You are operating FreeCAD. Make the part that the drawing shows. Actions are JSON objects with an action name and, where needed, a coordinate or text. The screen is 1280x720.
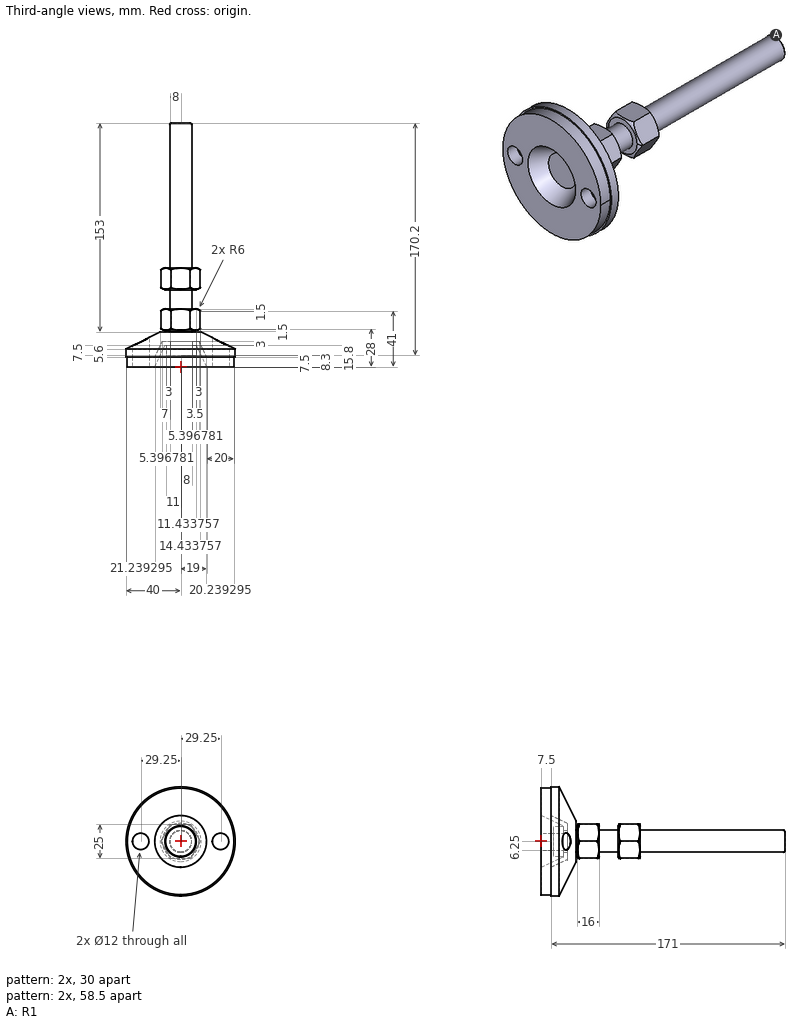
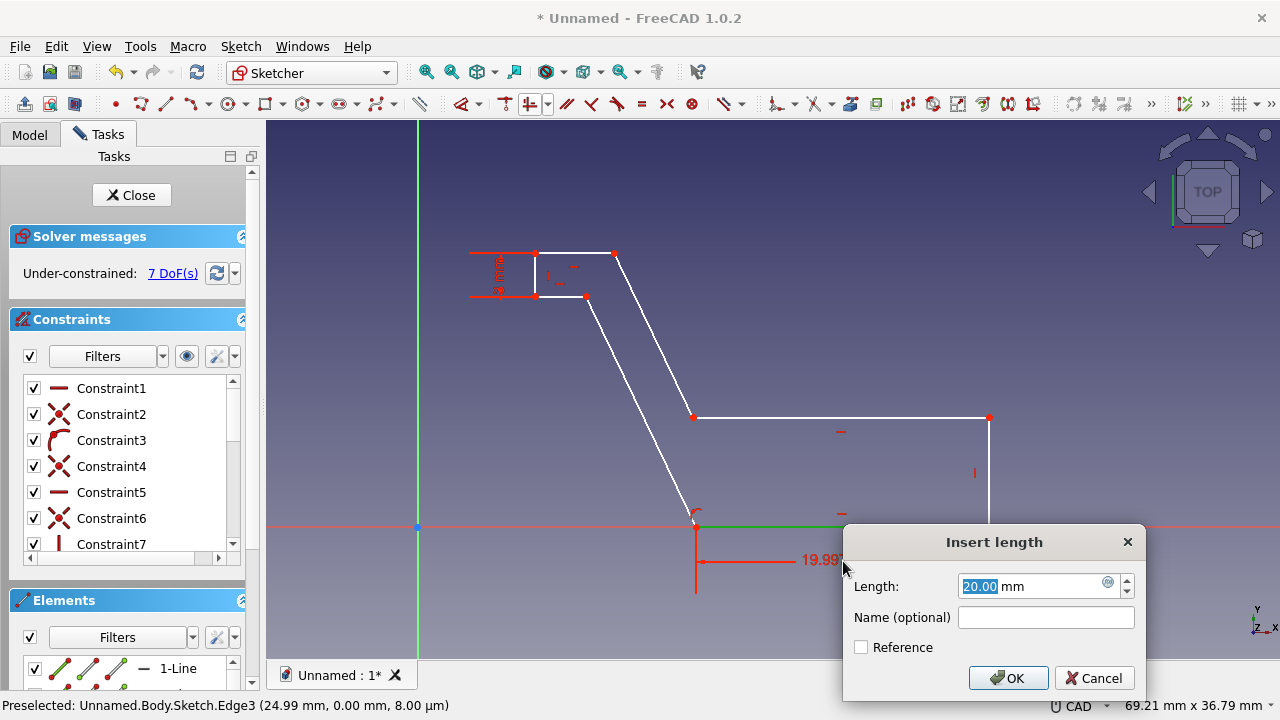
{"action": "type", "text": "20"}
{"action": "key", "text": "Return"}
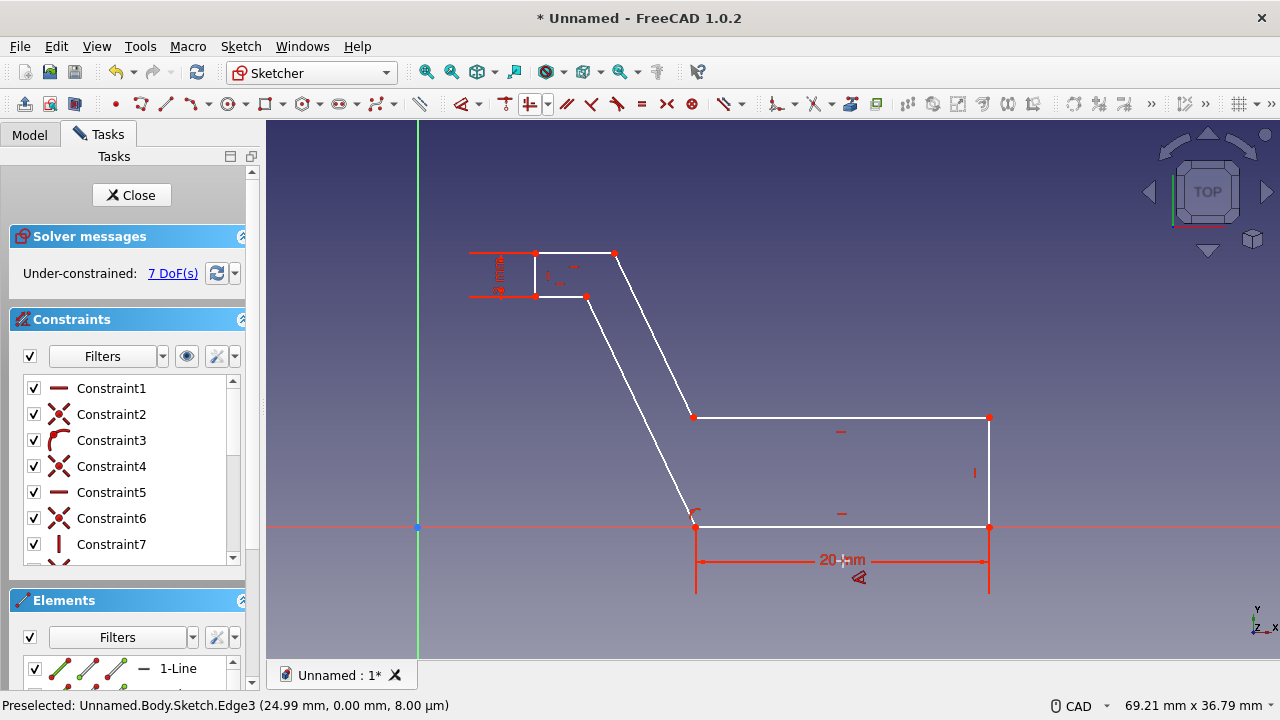
{"action": "left_click", "coordinate": [535, 297]}
{"action": "left_click", "coordinate": [476, 561]}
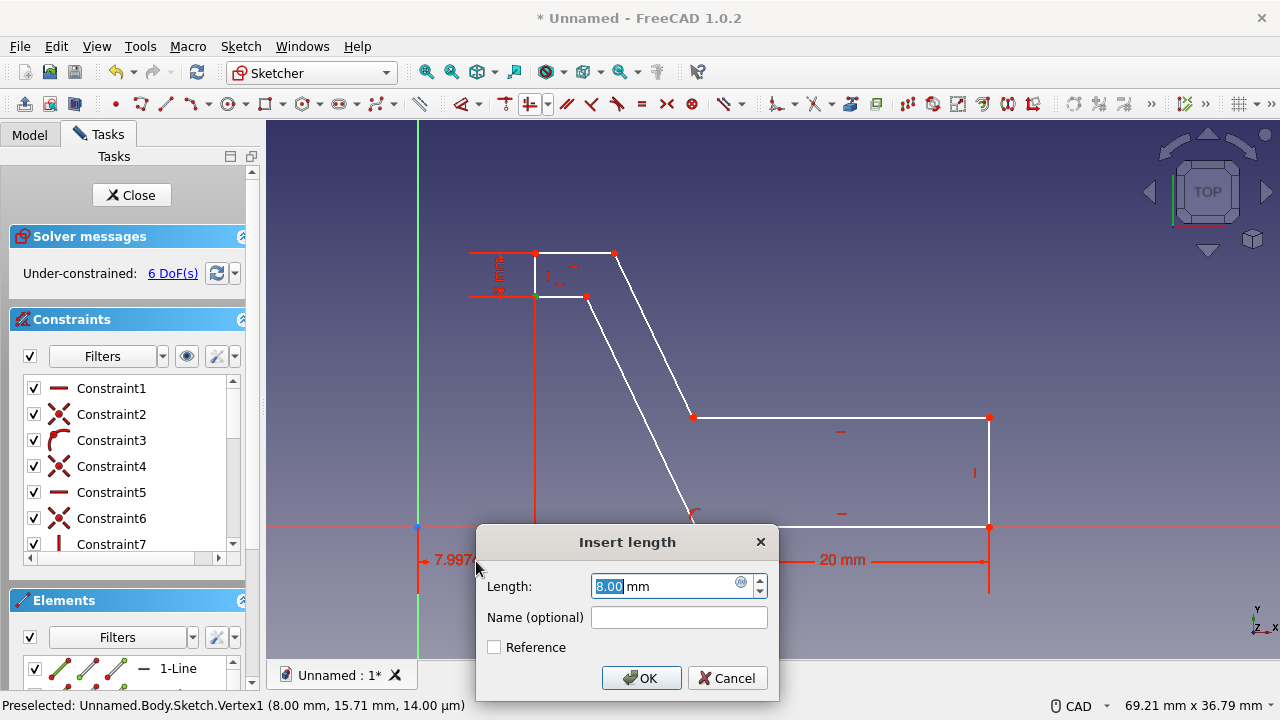
{"action": "type", "text": "8"}
{"action": "key", "text": "Return"}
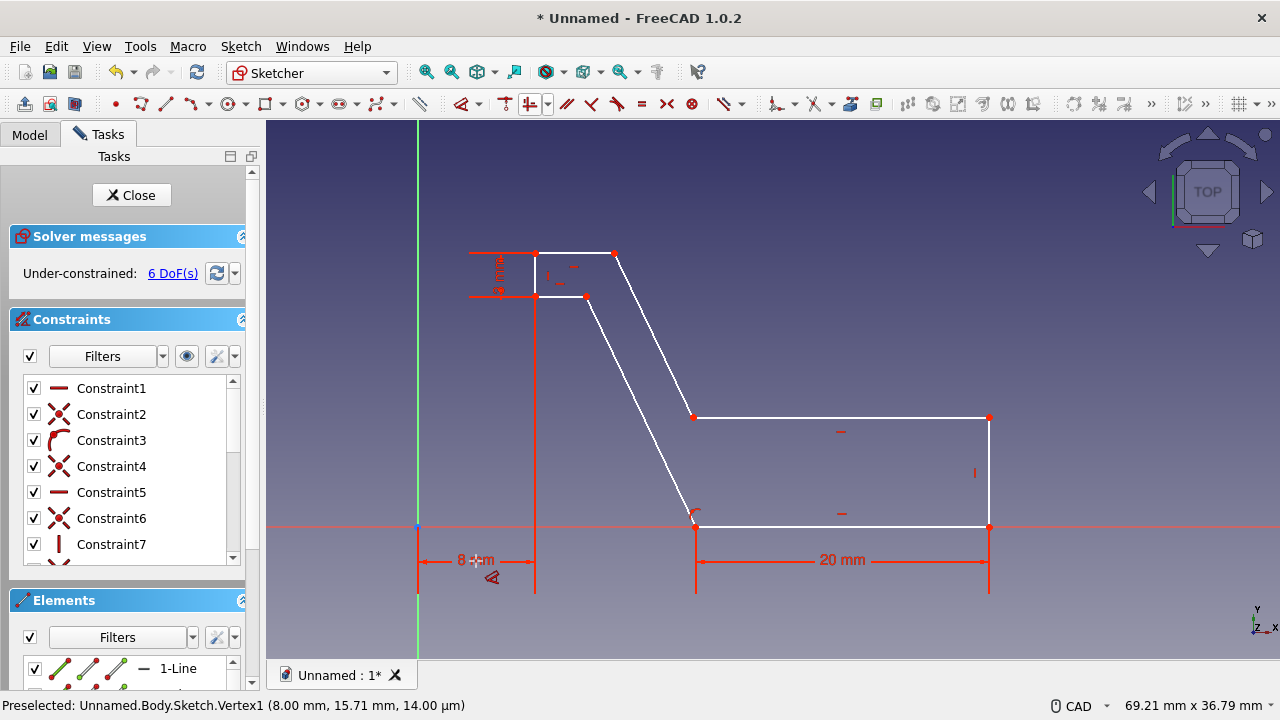
{"action": "left_click", "coordinate": [550, 297]}
{"action": "left_click", "coordinate": [561, 331]}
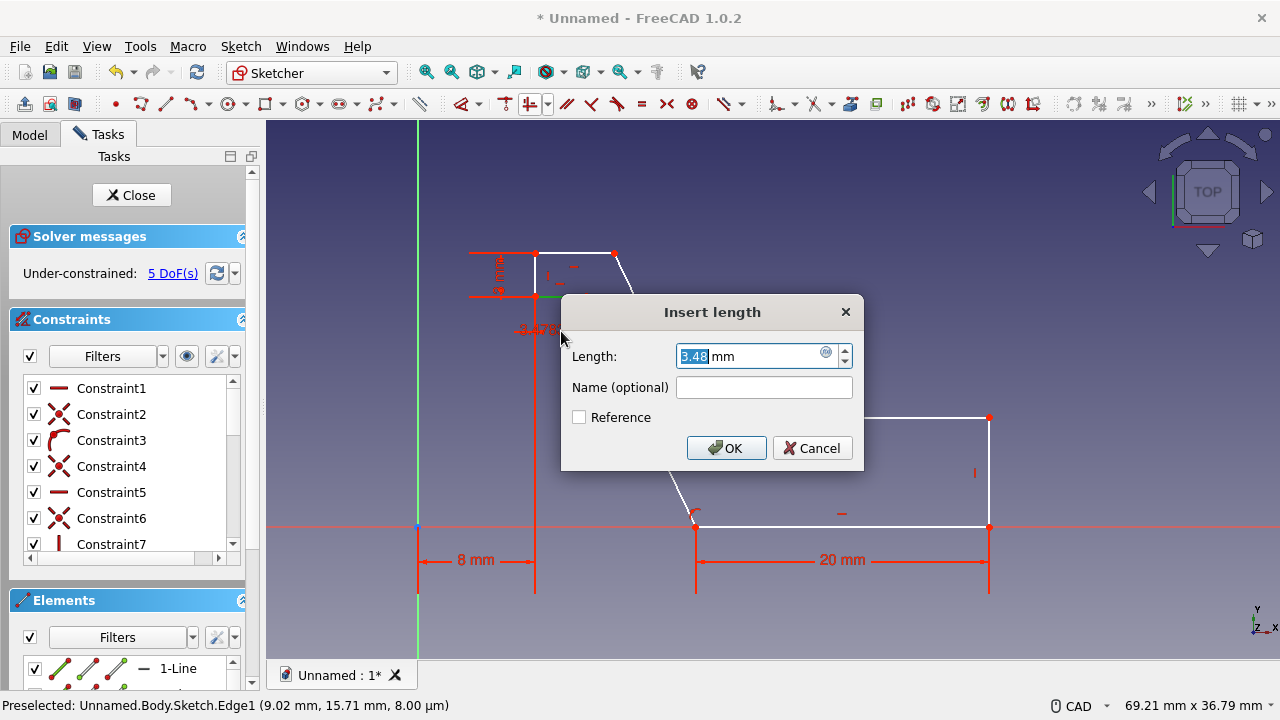
{"action": "type", "text": "3.5"}
{"action": "key", "text": "Return"}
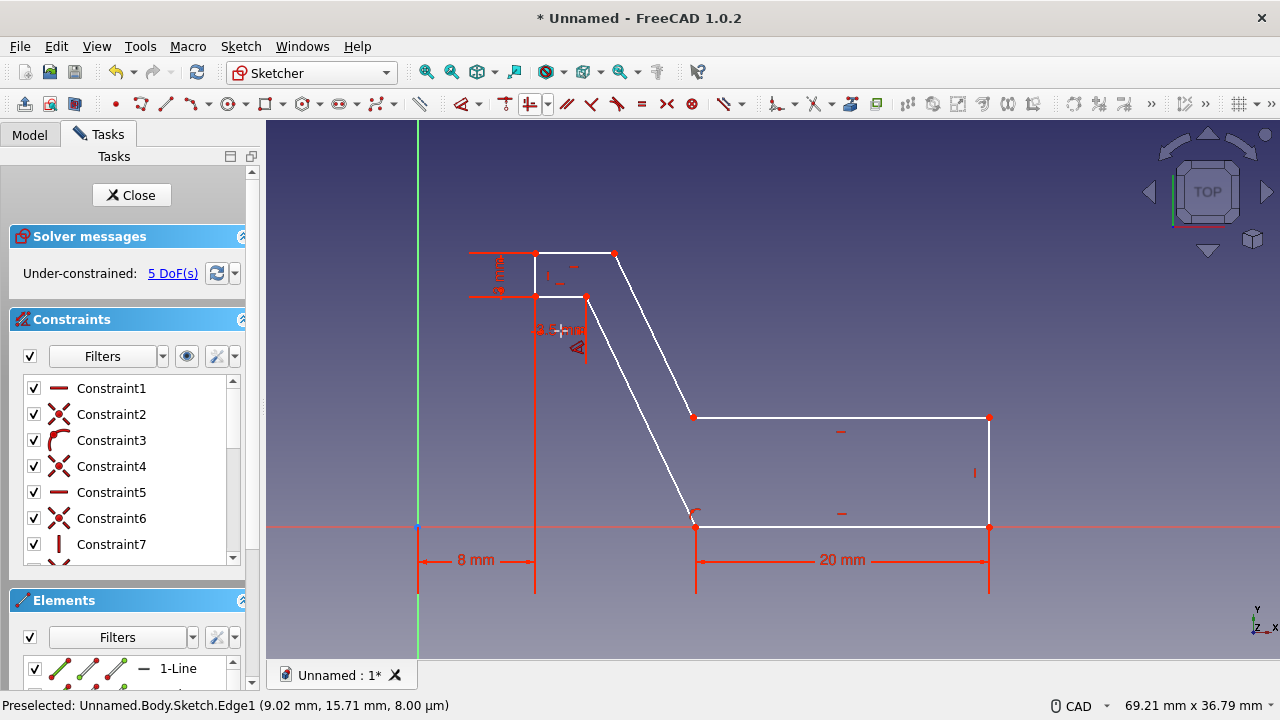
{"action": "left_click", "coordinate": [989, 494]}
{"action": "left_click", "coordinate": [1023, 473]}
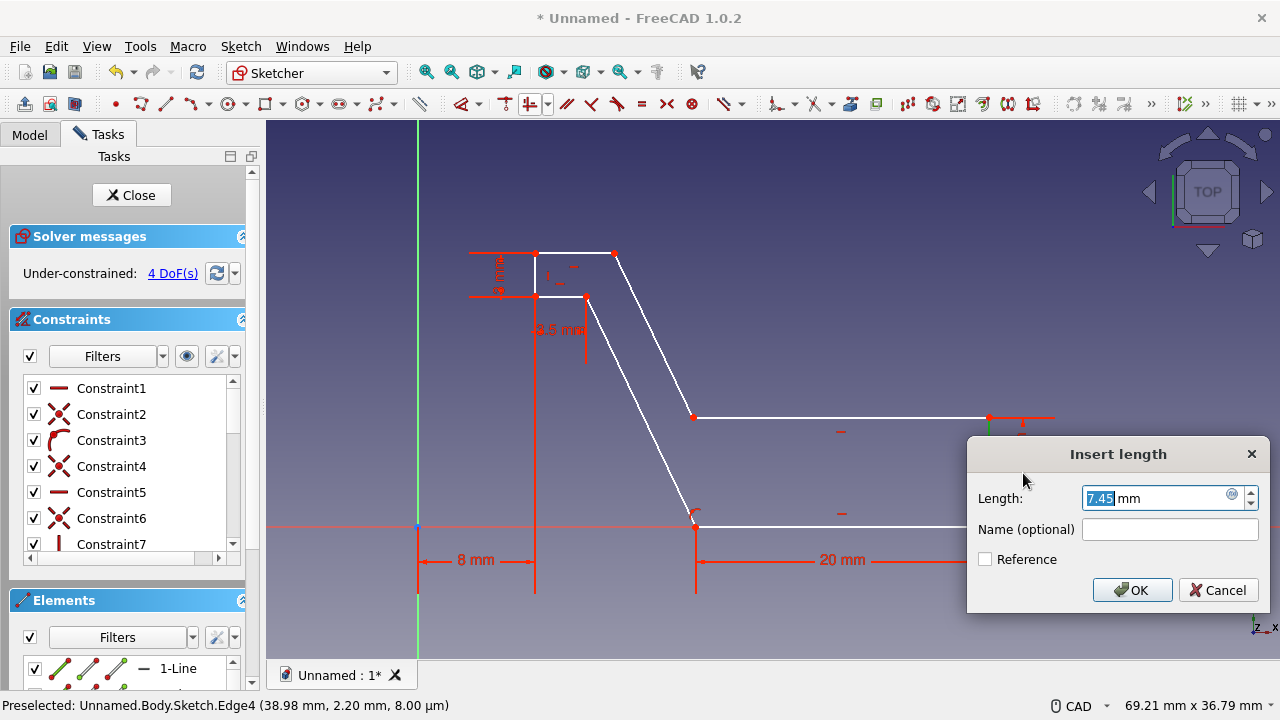
{"action": "type", "text": "7.5"}
{"action": "key", "text": "Return"}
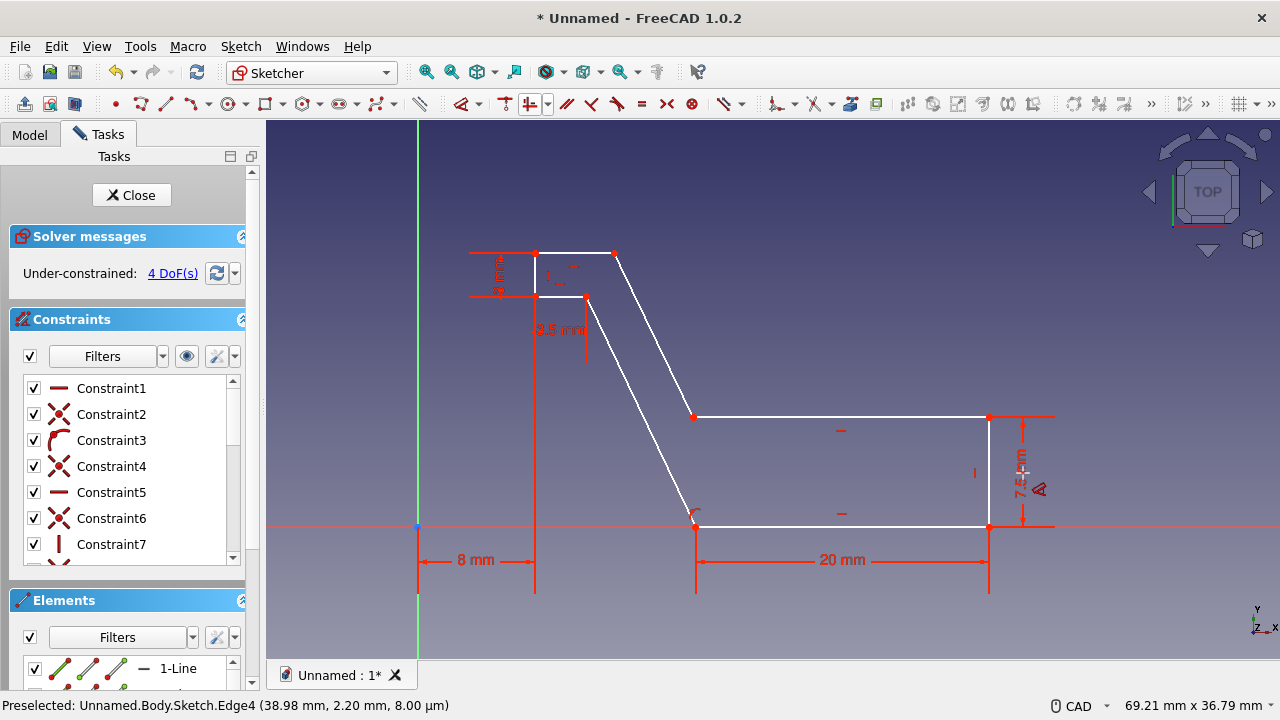
{"action": "left_click", "coordinate": [696, 527]}
{"action": "left_click", "coordinate": [557, 561]}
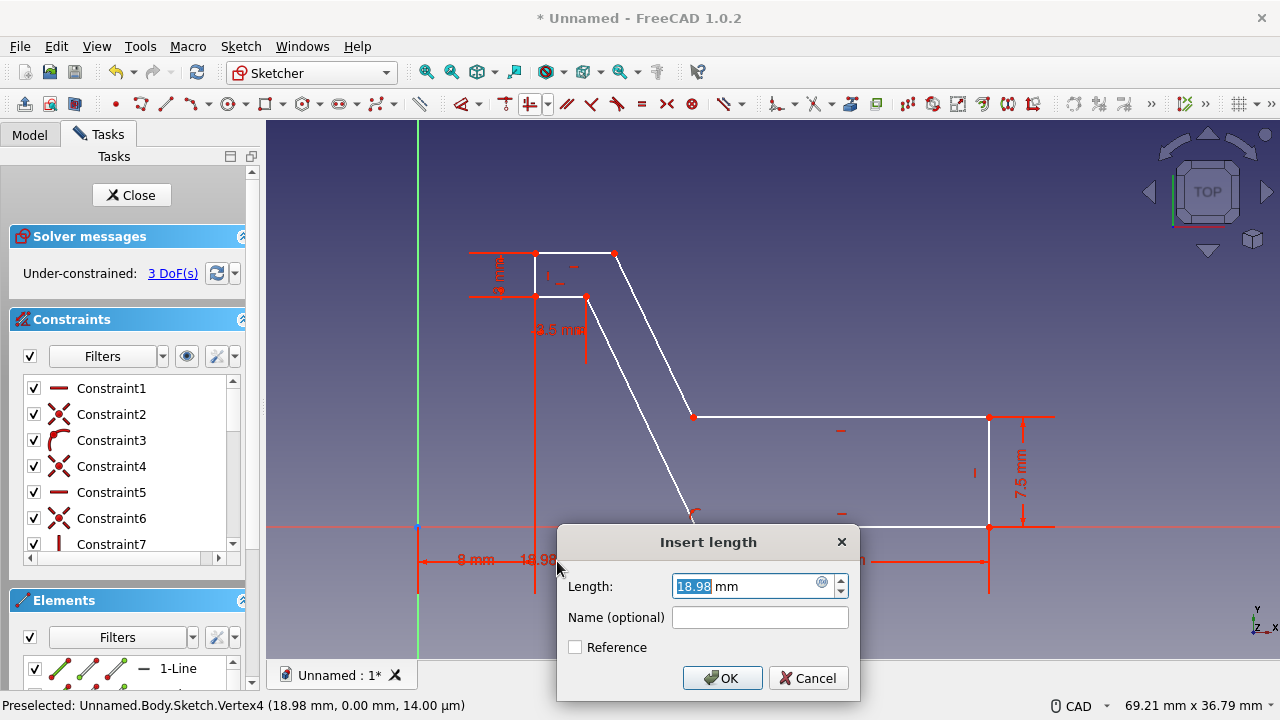
{"action": "type", "text": "19"}
{"action": "key", "text": "Return"}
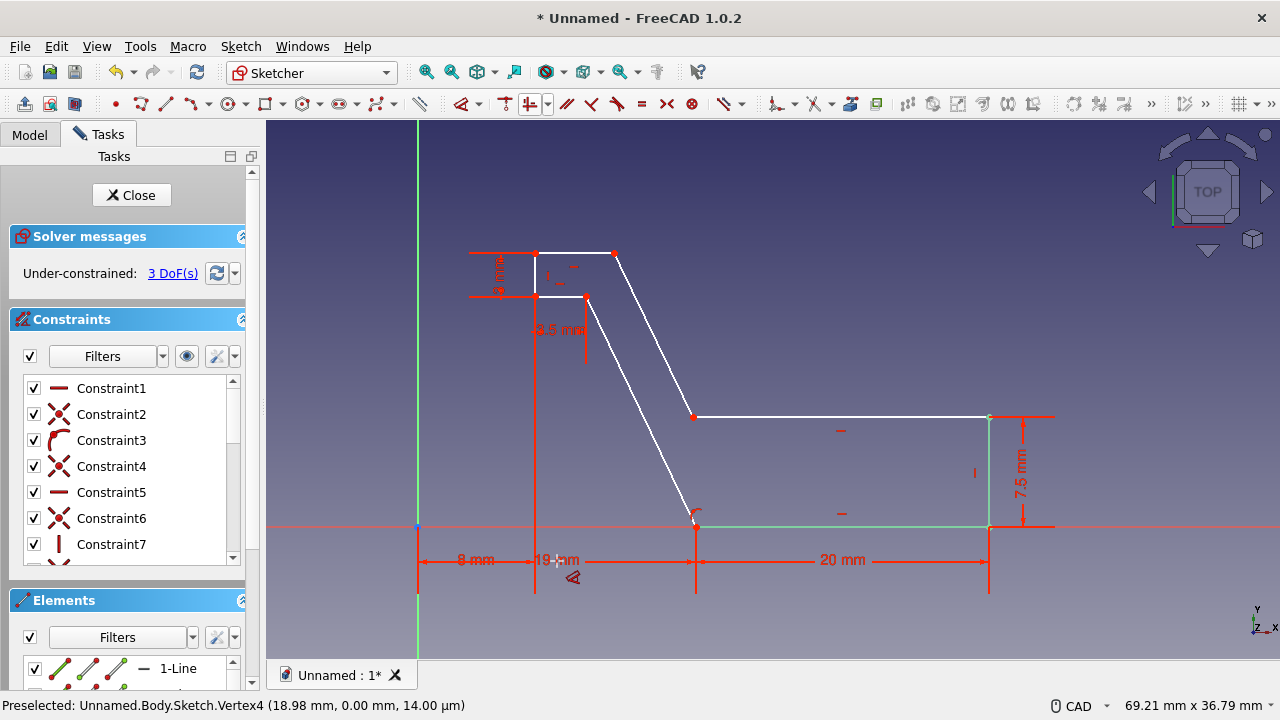
{"action": "left_click", "coordinate": [535, 297]}
{"action": "left_click", "coordinate": [384, 412]}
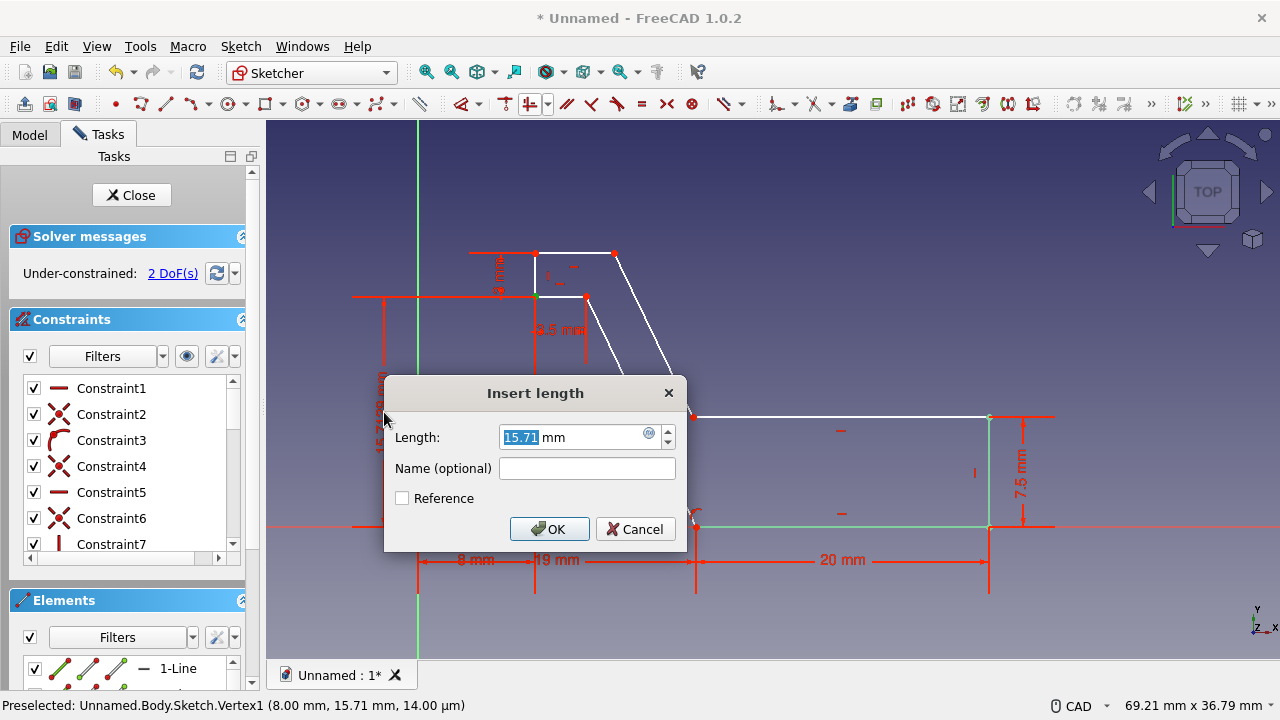
{"action": "type", "text": "15.8"}
{"action": "key", "text": "Return"}